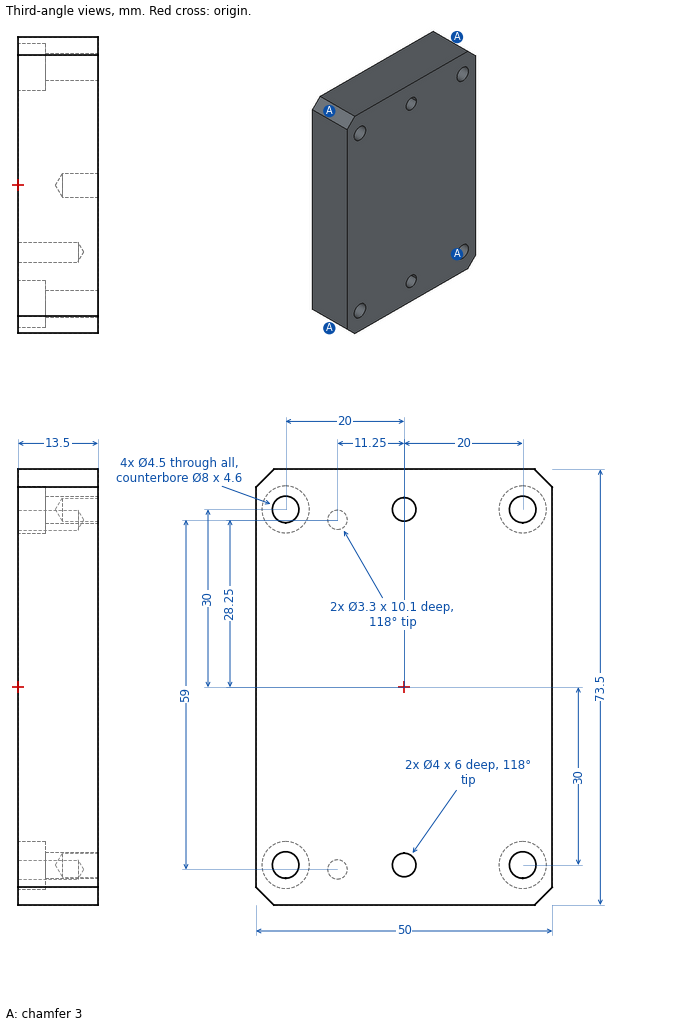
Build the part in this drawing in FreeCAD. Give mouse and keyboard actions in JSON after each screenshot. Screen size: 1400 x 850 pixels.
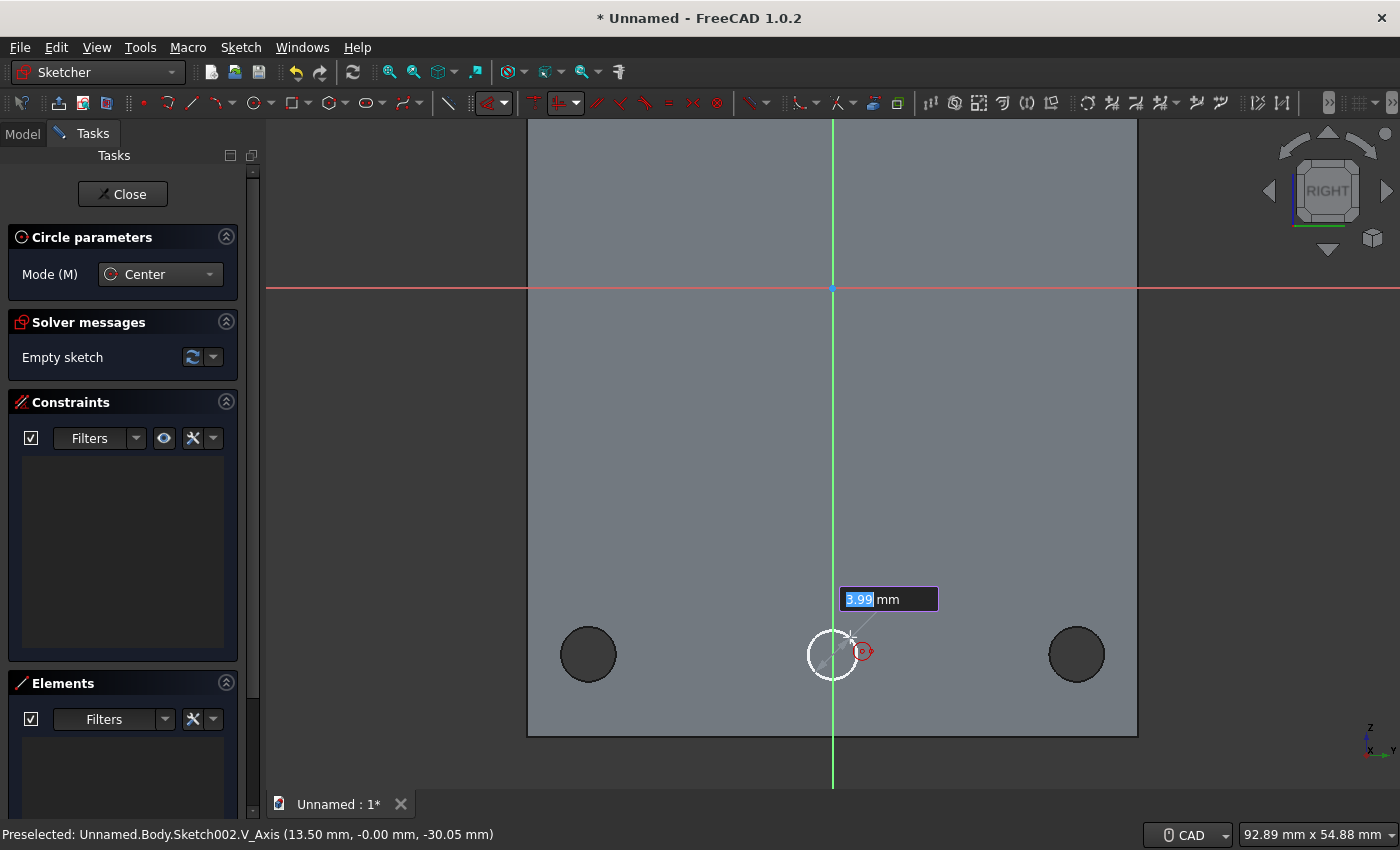
{"action": "type", "text": "4"}
{"action": "key", "text": "Return"}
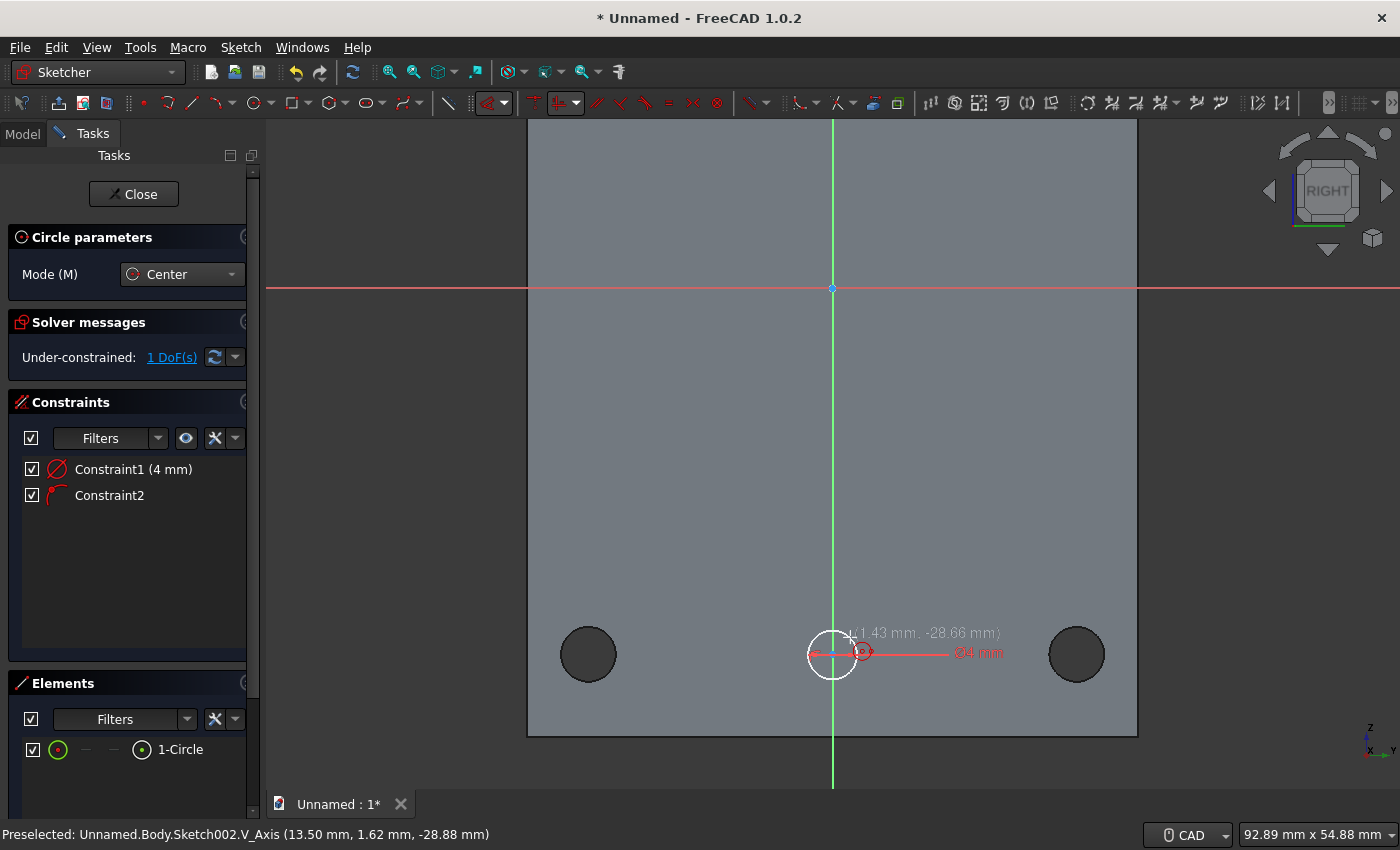
{"action": "scroll", "coordinate": [682, 656], "scroll_direction": "down", "scroll_amount": 3}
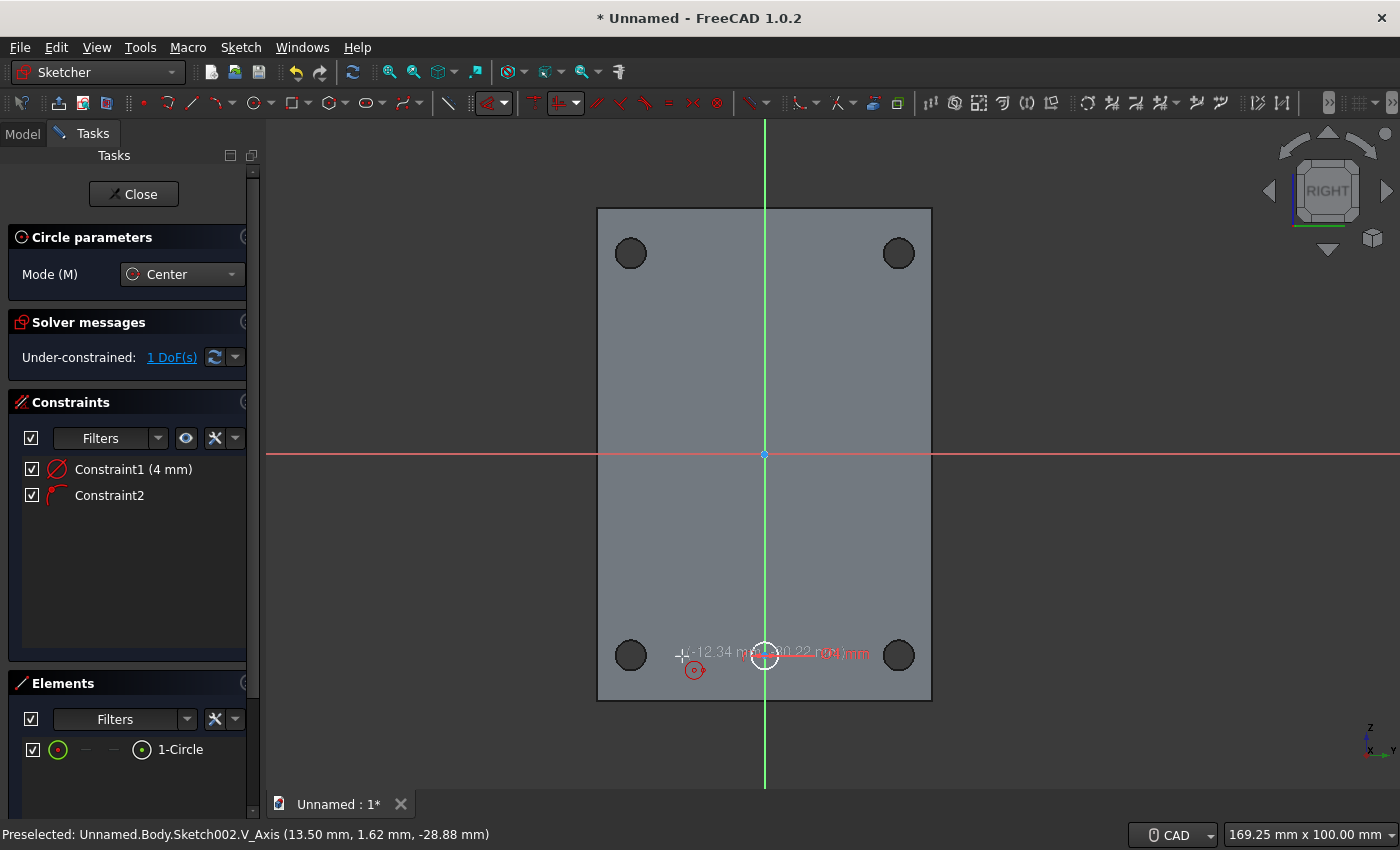
{"action": "scroll", "coordinate": [765, 253], "scroll_direction": "up", "scroll_amount": 3}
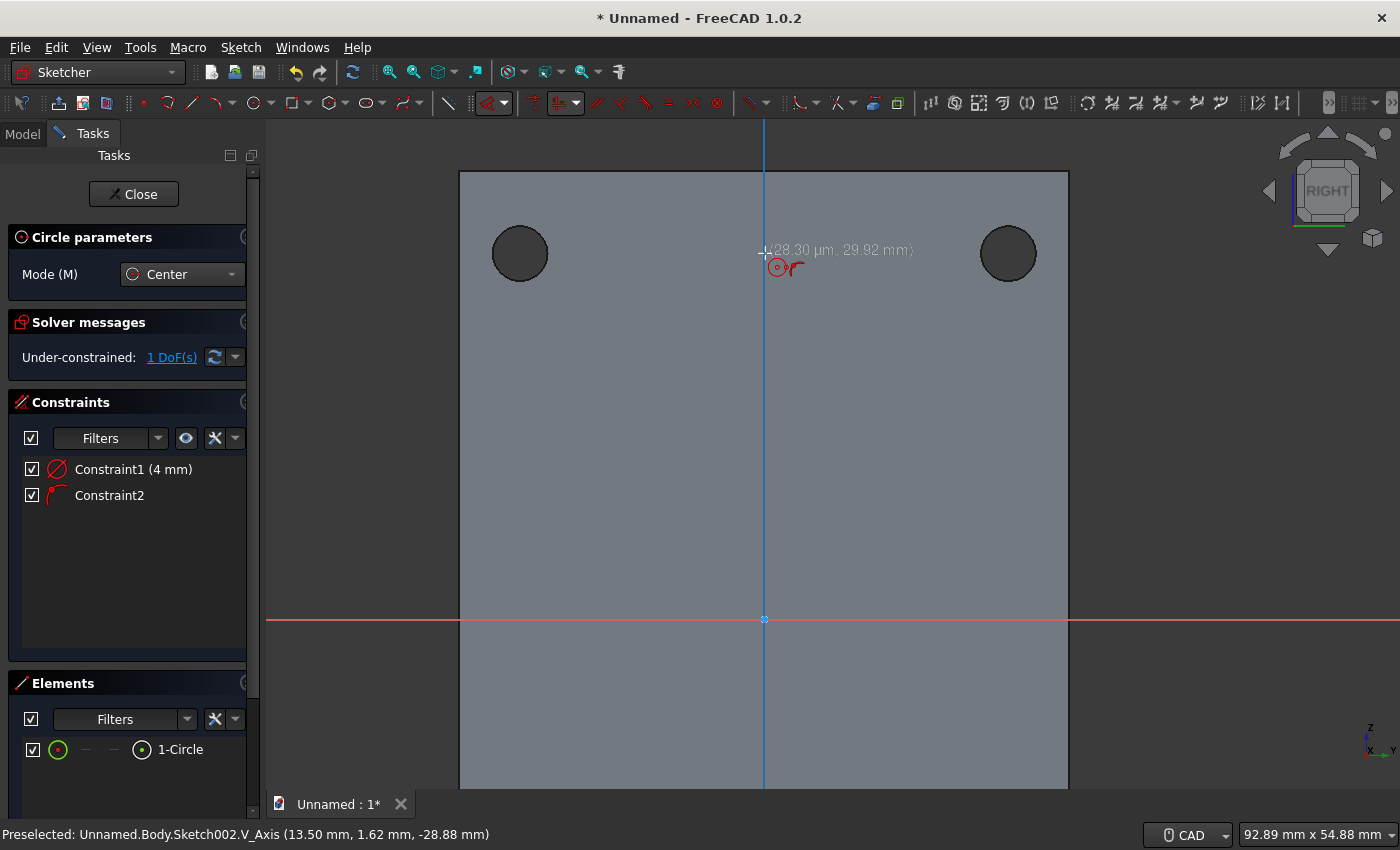
{"action": "left_click", "coordinate": [764, 254]}
{"action": "mouse_move", "coordinate": [782, 236]}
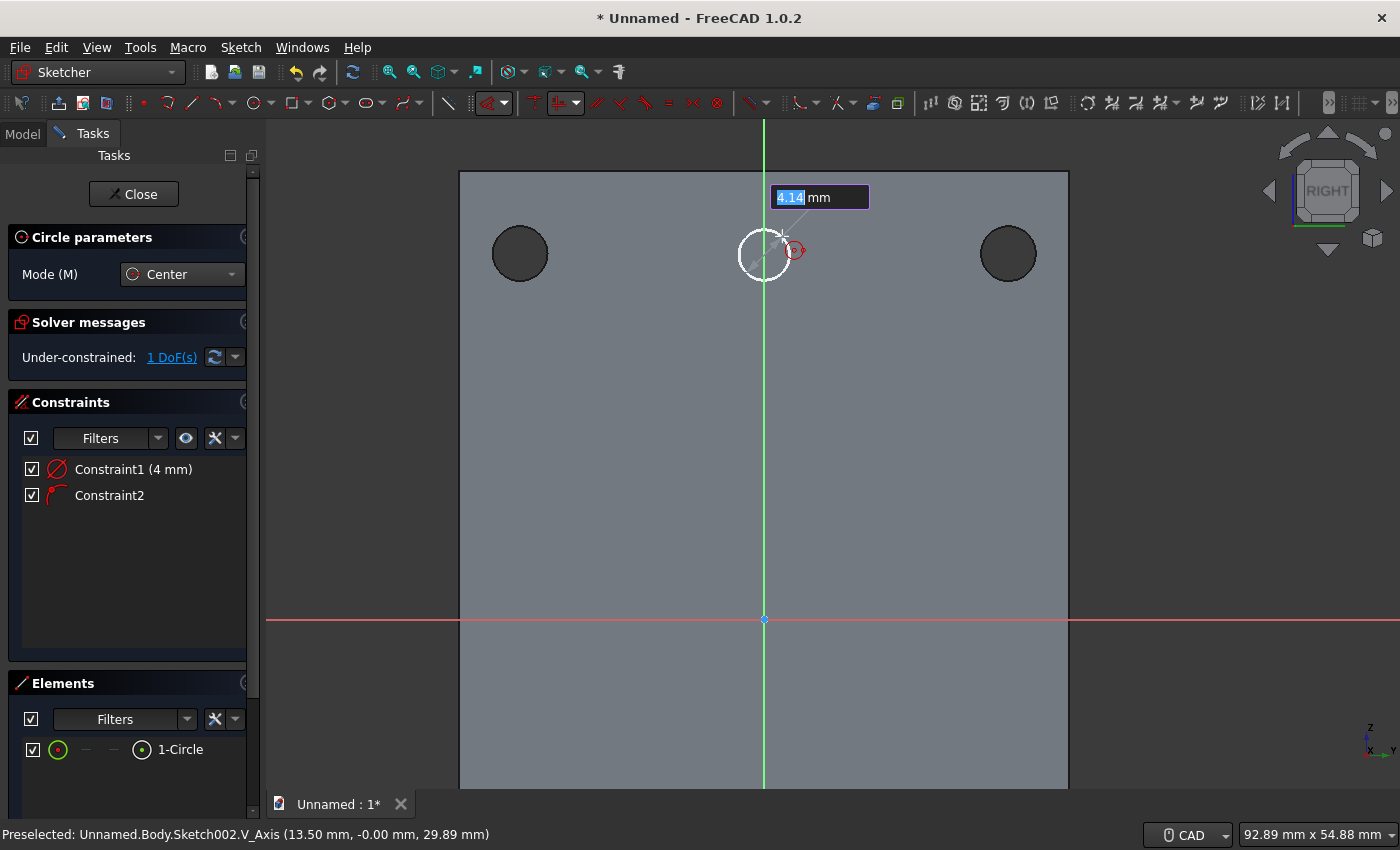
{"action": "type", "text": "4"}
{"action": "key", "text": "Return"}
{"action": "key", "text": "Escape"}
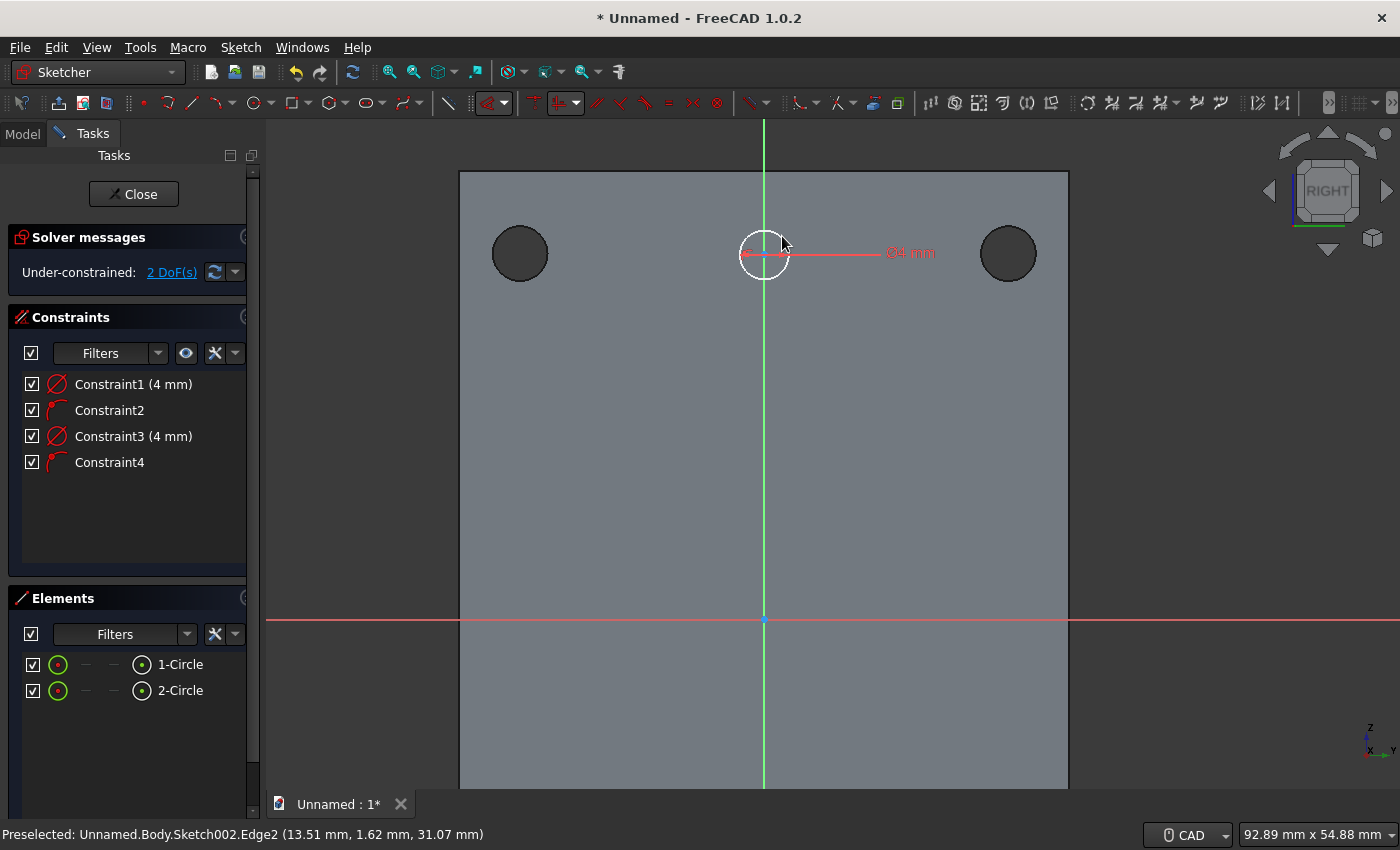
{"action": "scroll", "coordinate": [765, 252], "scroll_direction": "down", "scroll_amount": 3}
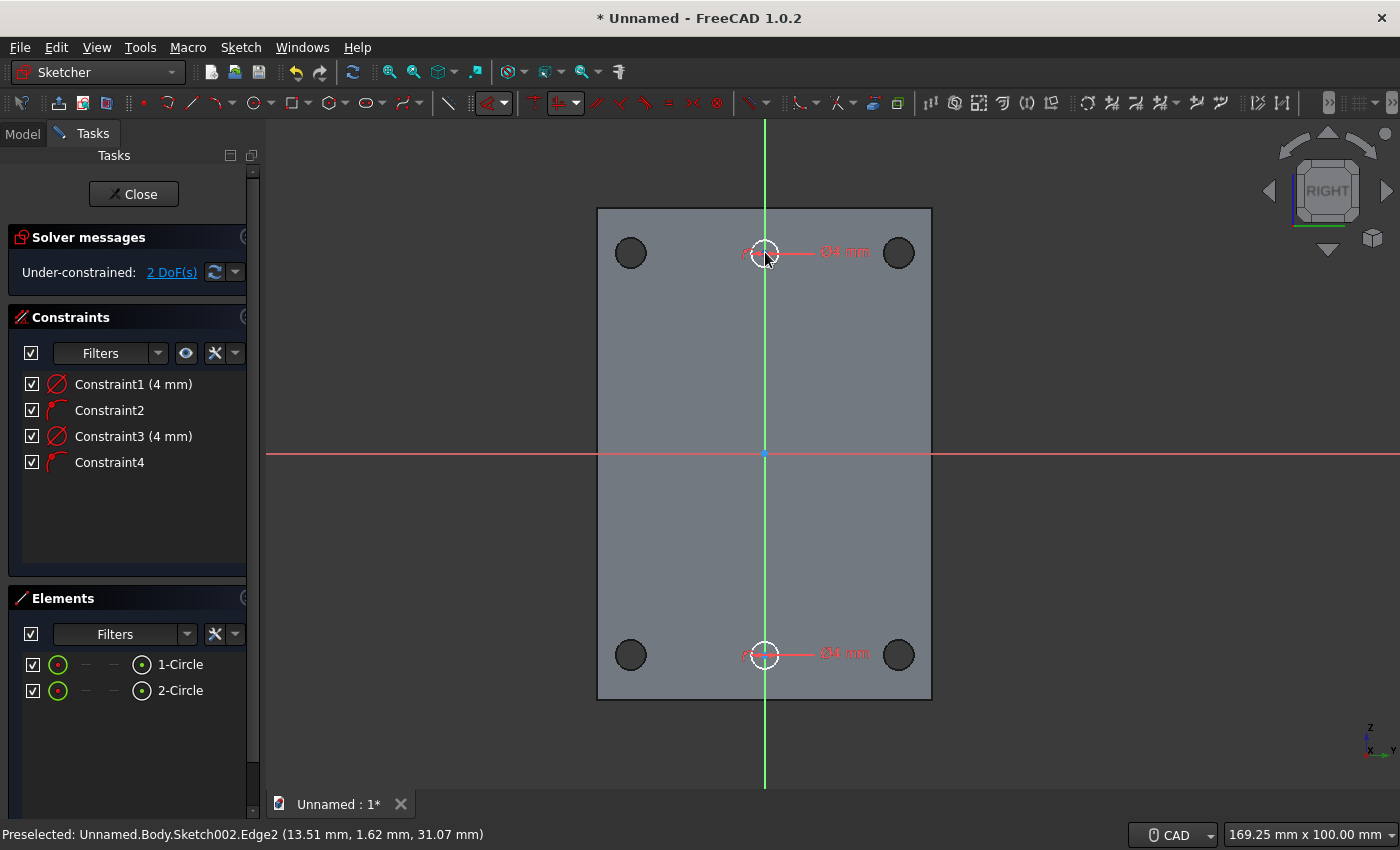
{"action": "left_click", "coordinate": [765, 655]}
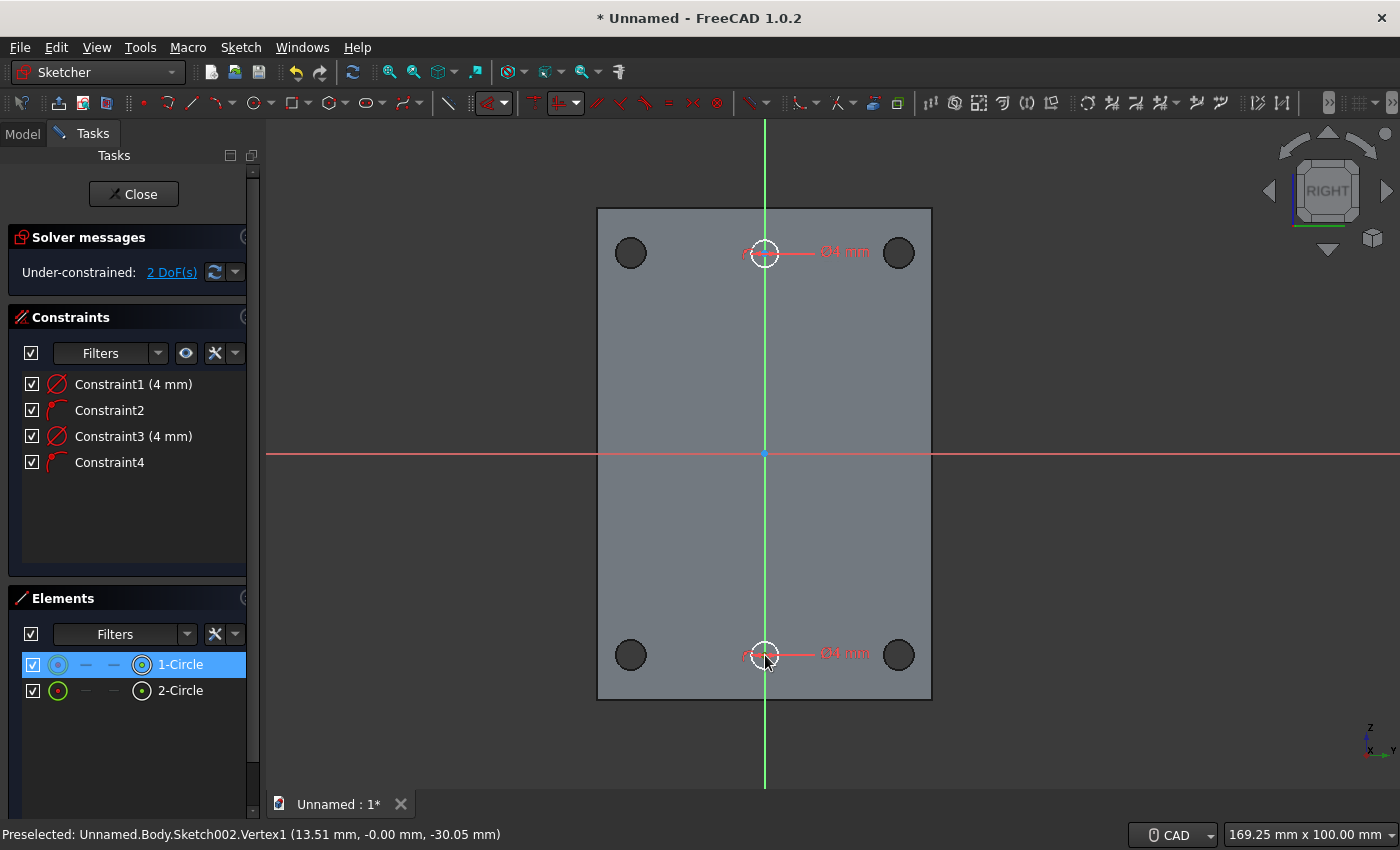
{"action": "left_click", "coordinate": [506, 104]}